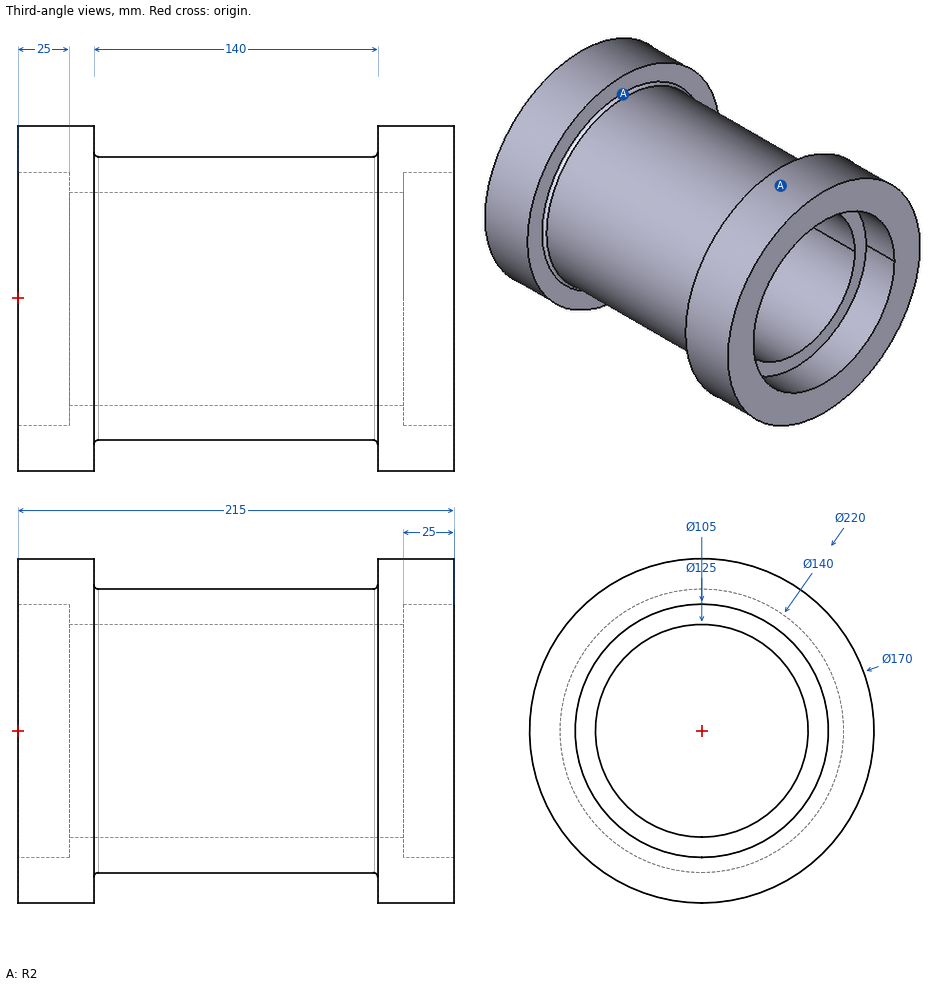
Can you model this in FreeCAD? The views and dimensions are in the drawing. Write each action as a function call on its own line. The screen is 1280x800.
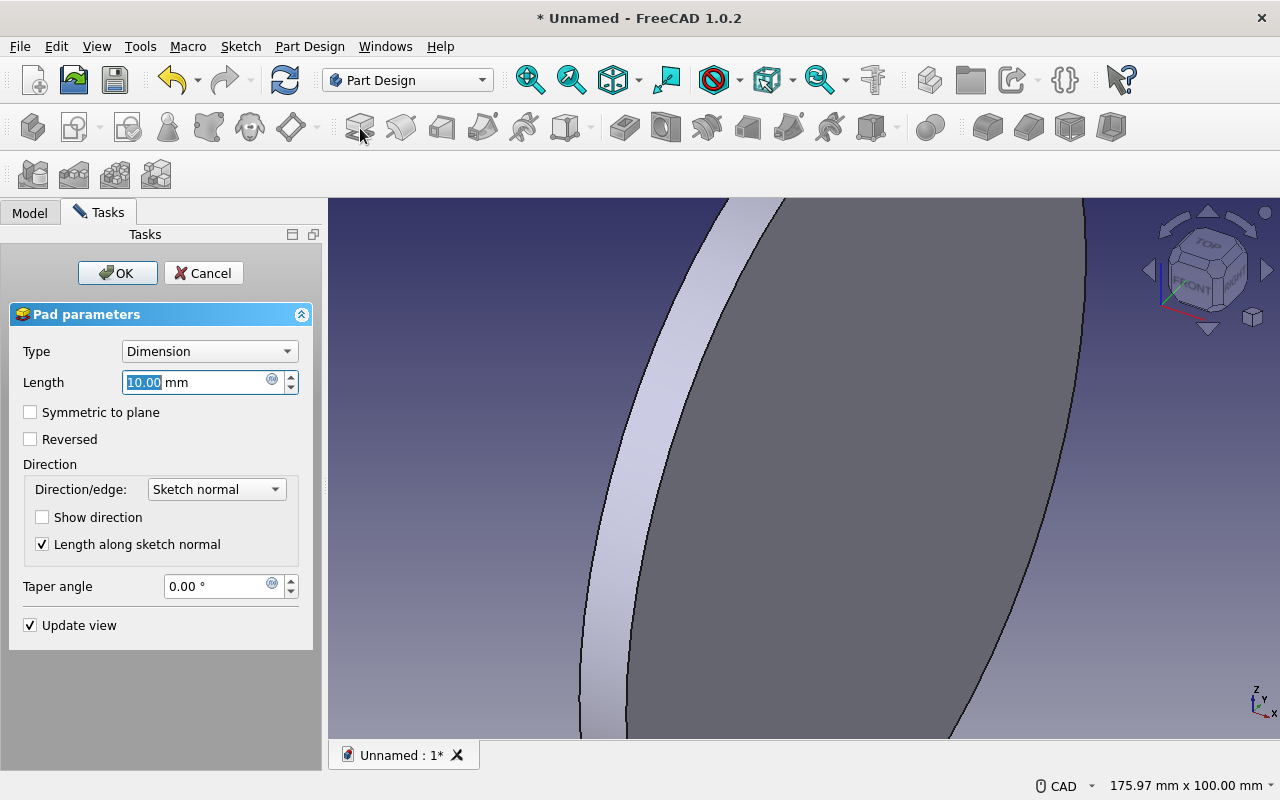
text(215)
key(Tab)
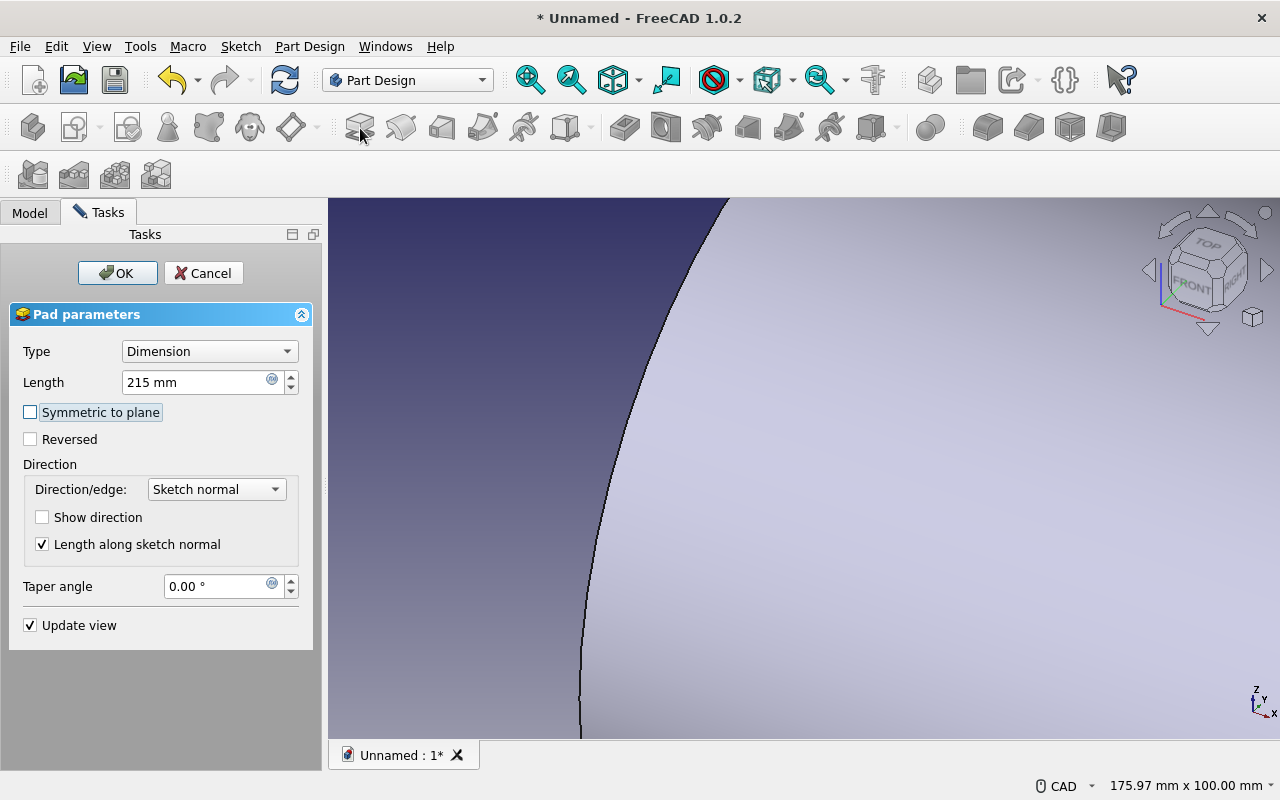
click(118, 273)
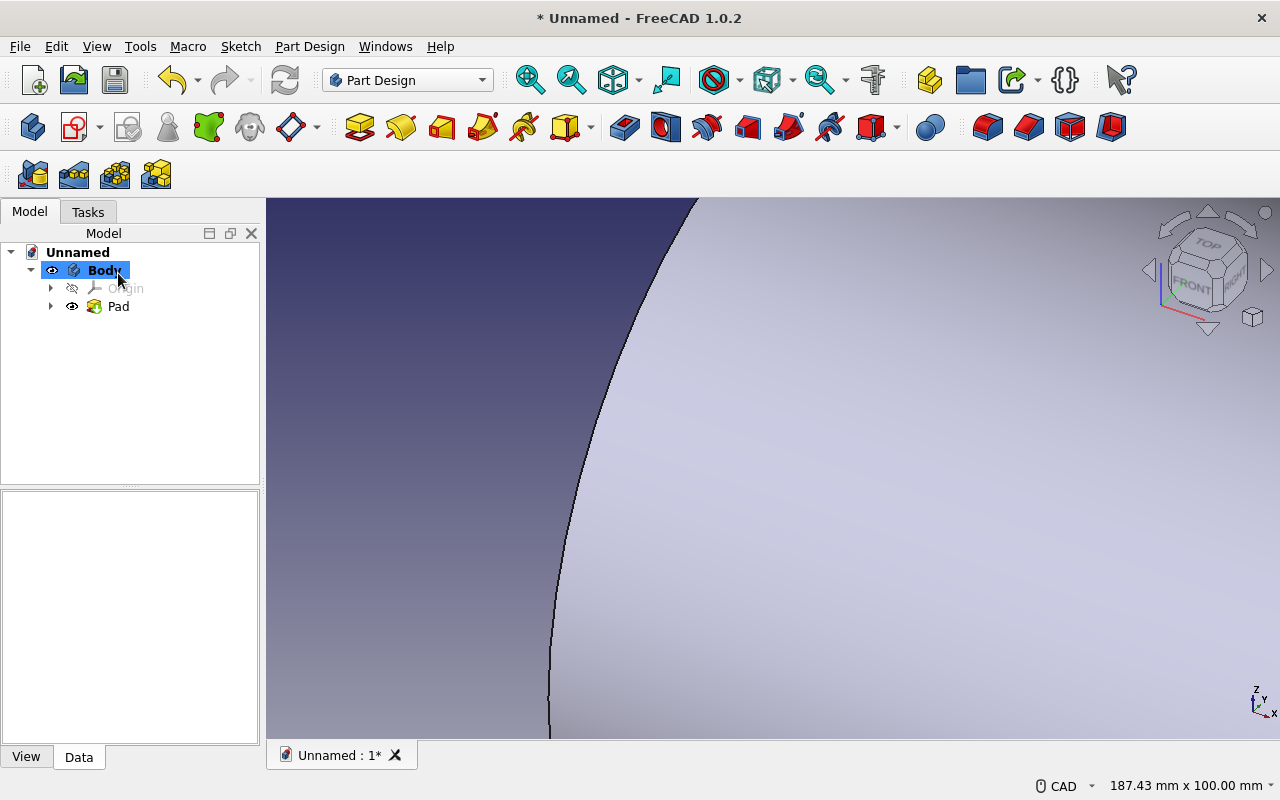
click(531, 80)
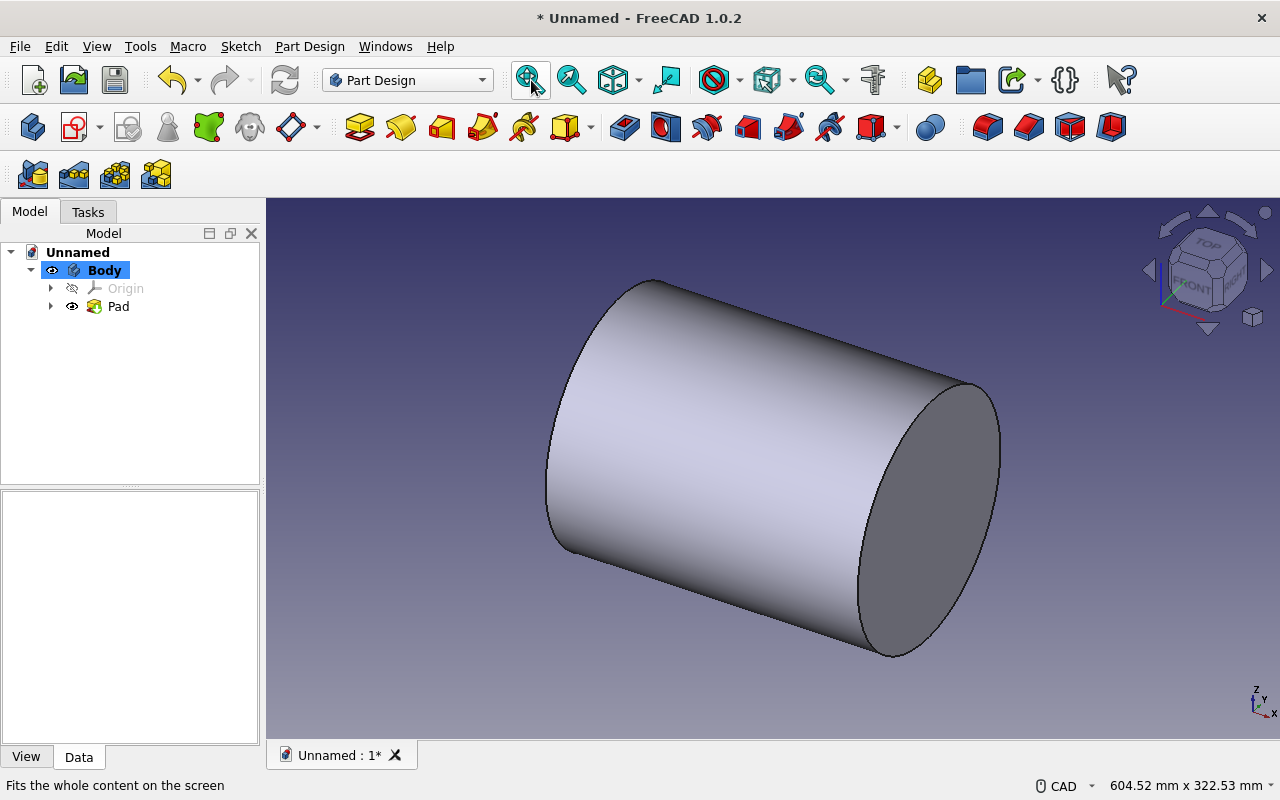
click(51, 288)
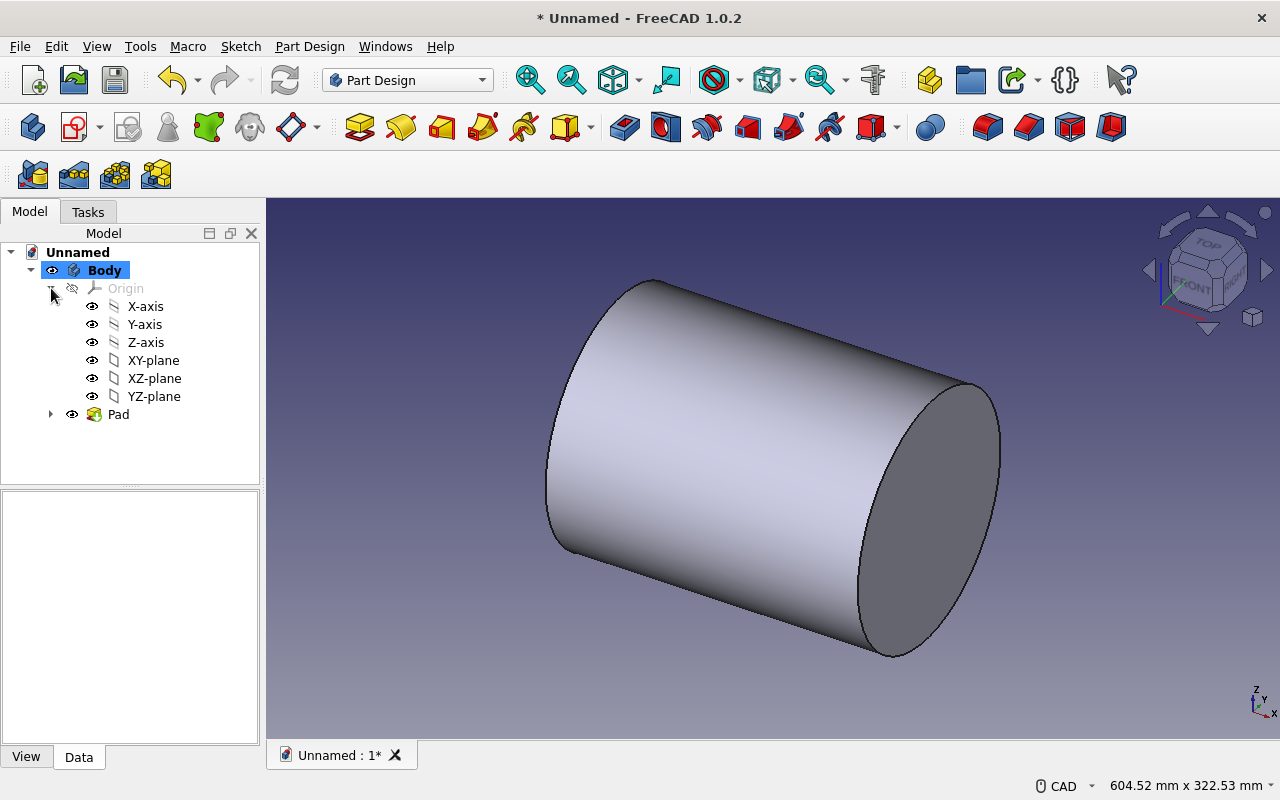
click(137, 396)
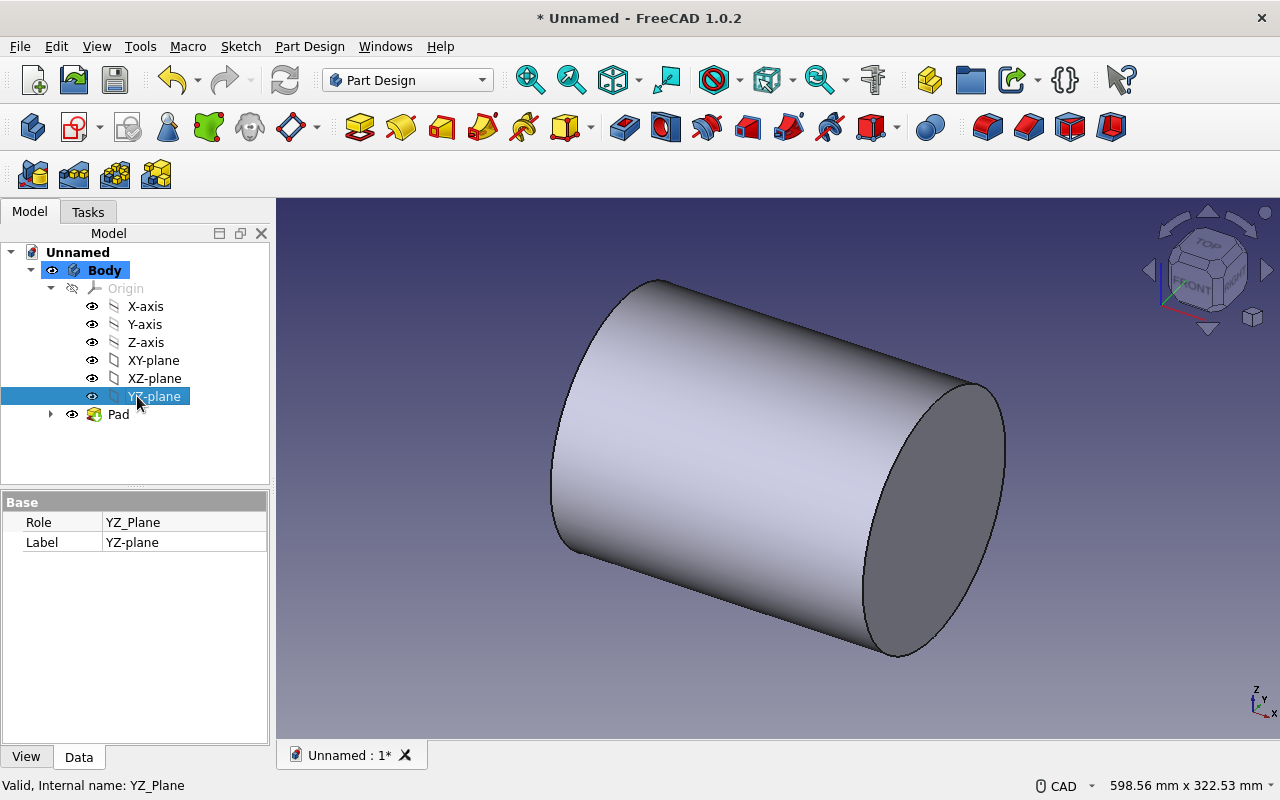
click(290, 128)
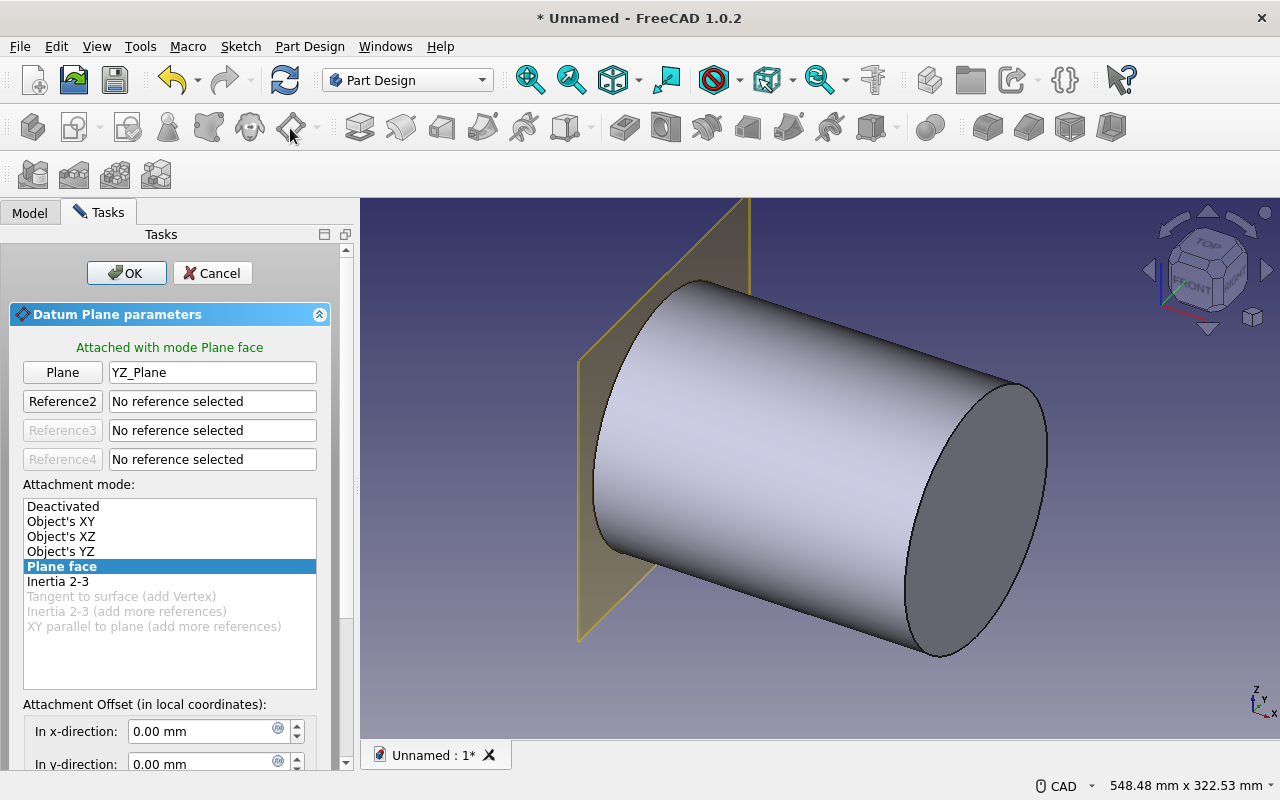
scroll(346, 507, down, 2)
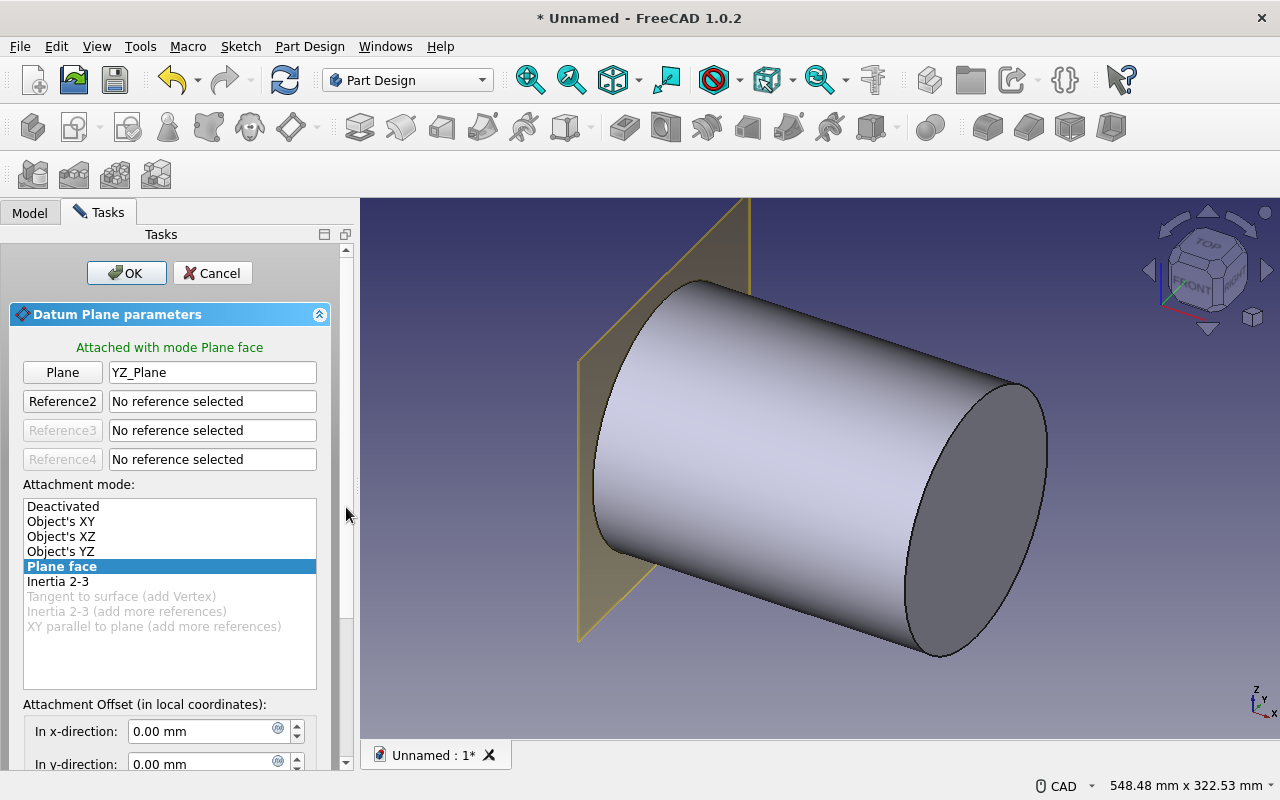
triple_click(210, 678)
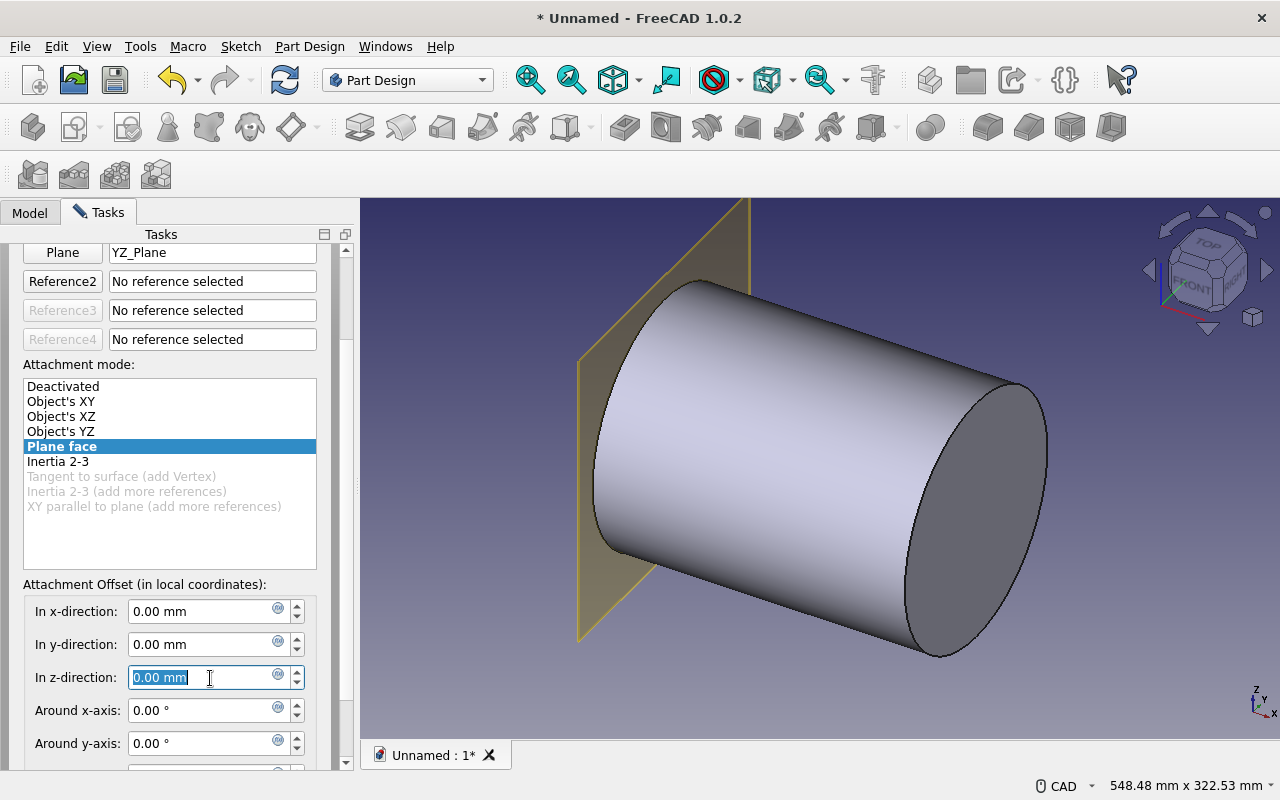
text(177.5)
key(Tab)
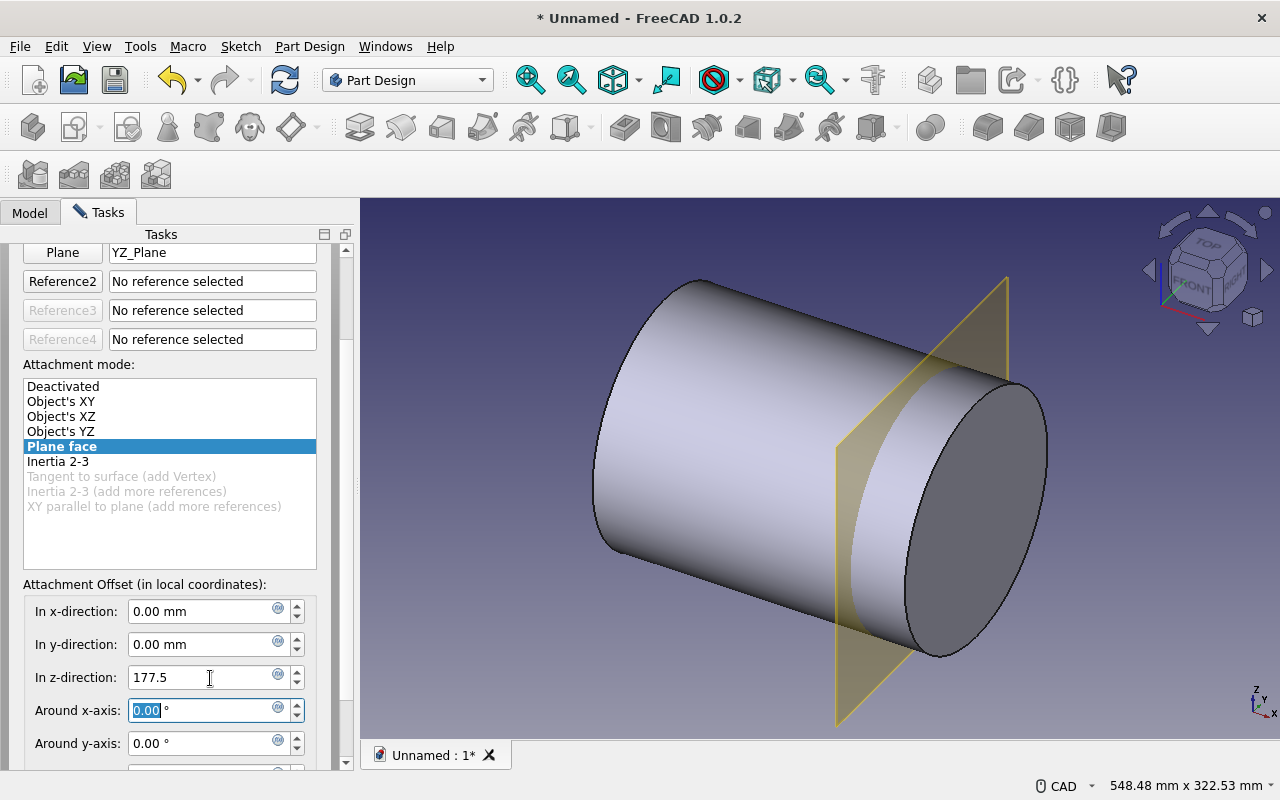
scroll(346, 507, up, 3)